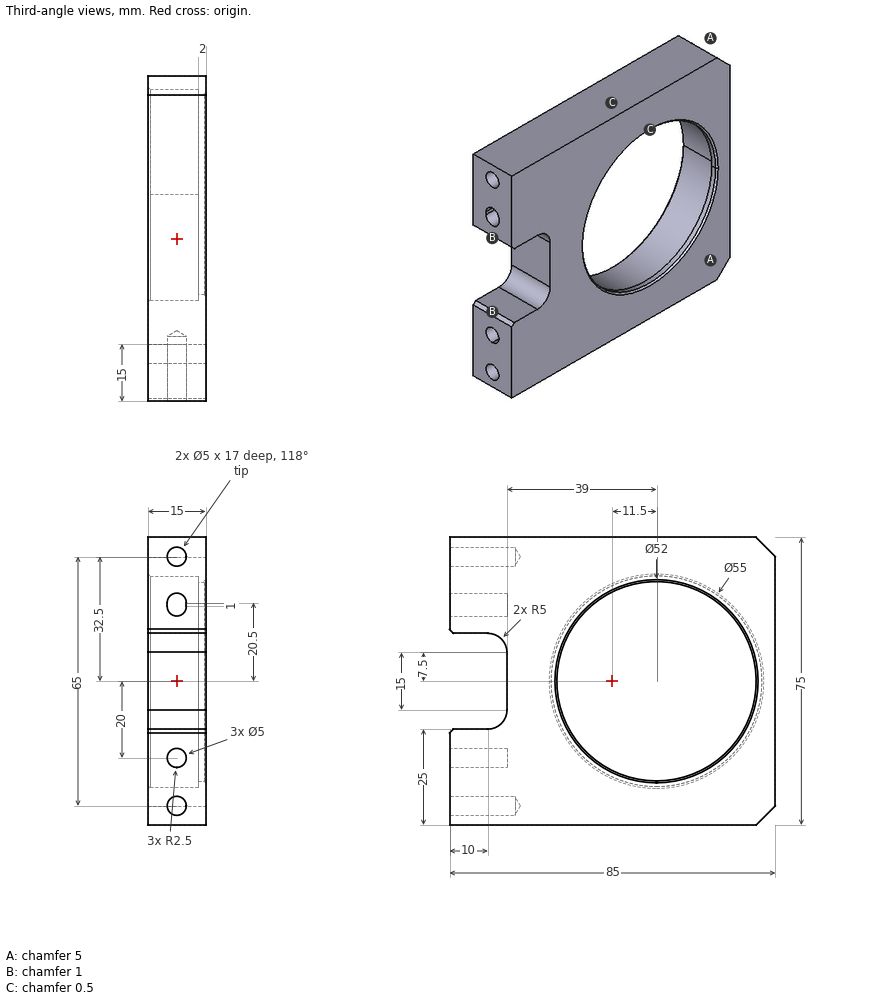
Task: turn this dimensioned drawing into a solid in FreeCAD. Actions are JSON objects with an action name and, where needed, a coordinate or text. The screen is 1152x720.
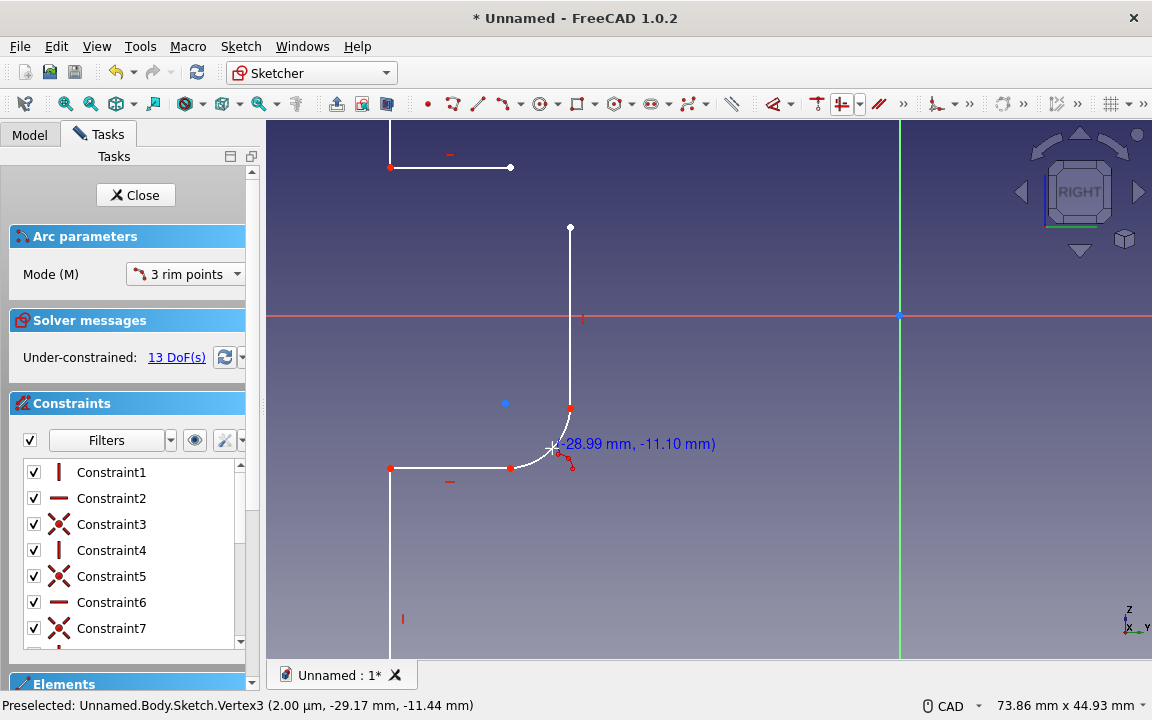
{"action": "left_click", "coordinate": [510, 168]}
{"action": "left_click", "coordinate": [570, 228]}
{"action": "left_click", "coordinate": [552, 183]}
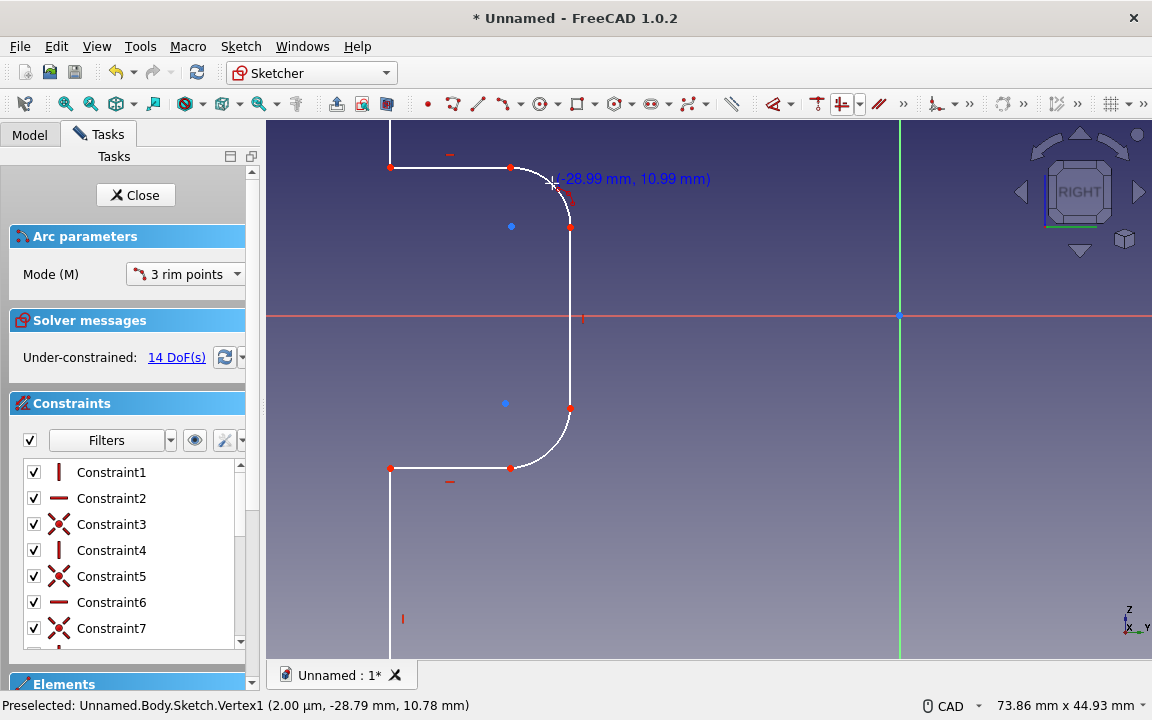
{"action": "left_click", "coordinate": [540, 104]}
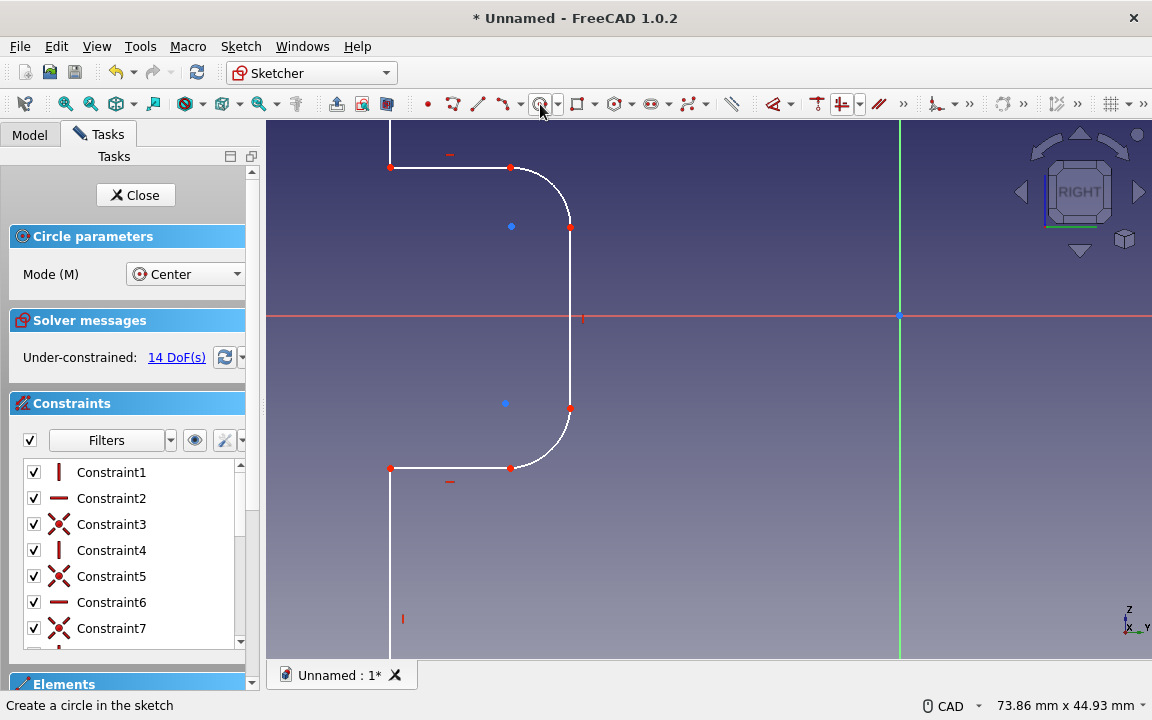
{"action": "scroll", "coordinate": [490, 432], "scroll_direction": "down", "scroll_amount": 5}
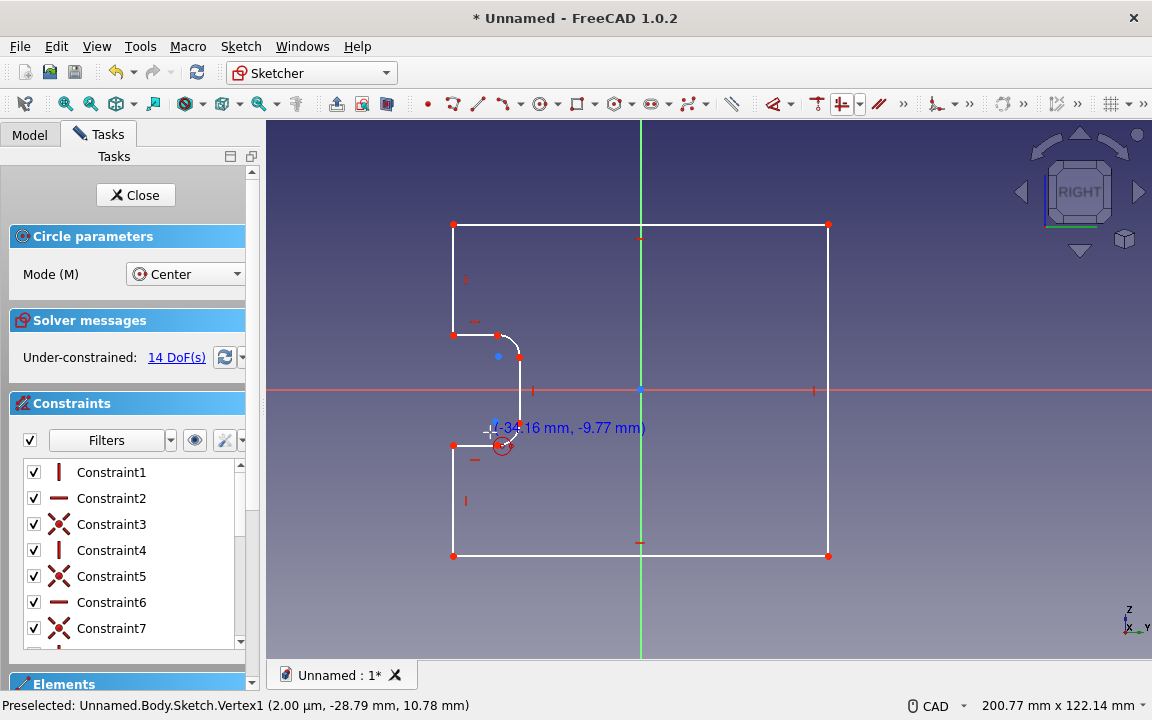
{"action": "left_click", "coordinate": [692, 390]}
{"action": "mouse_move", "coordinate": [777, 304]}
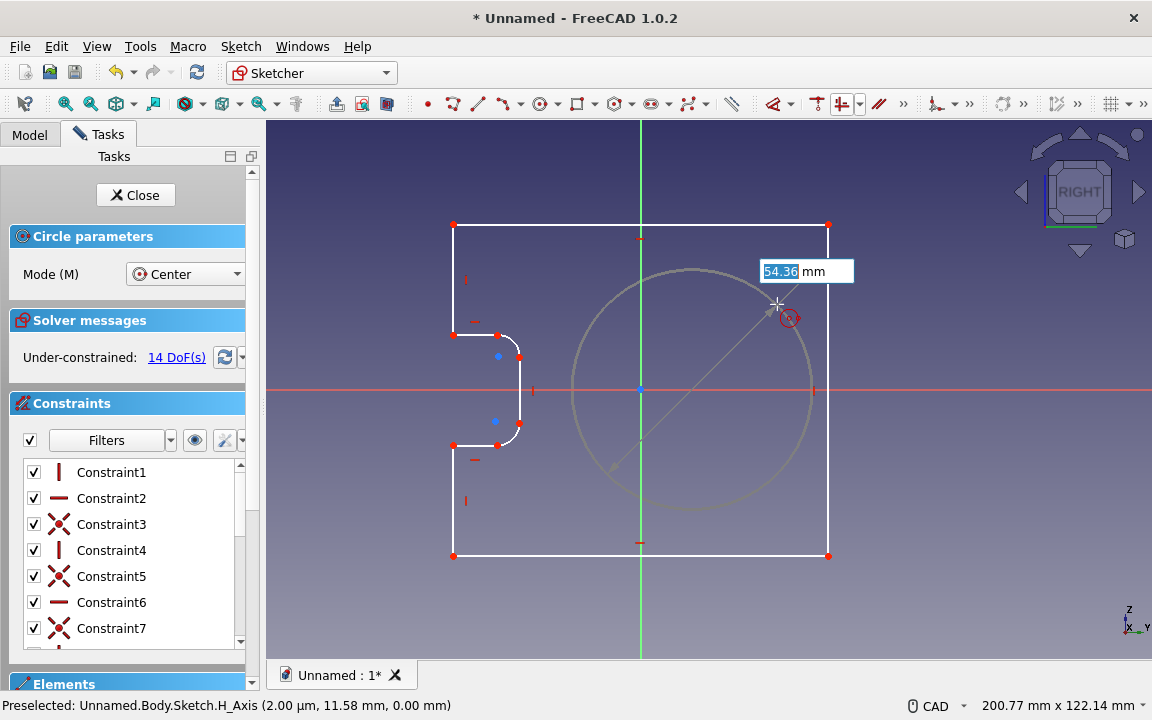
{"action": "type", "text": "55"}
{"action": "key", "text": "Return"}
{"action": "key", "text": "Escape"}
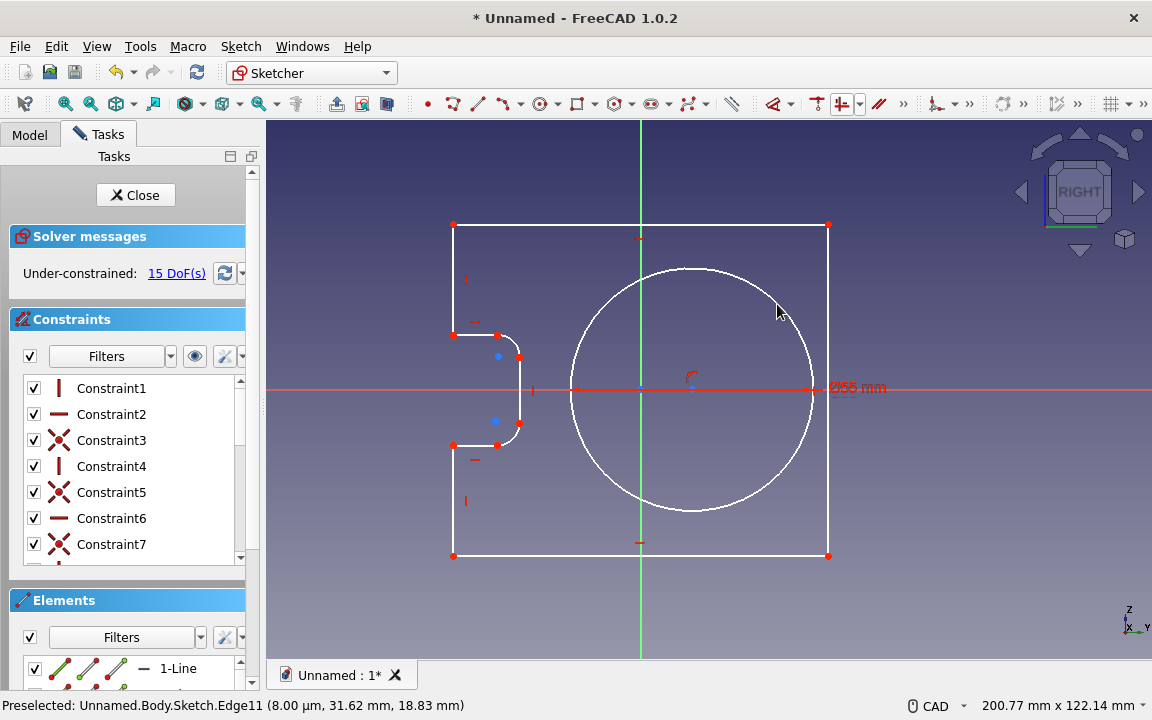
{"action": "left_click", "coordinate": [520, 377]}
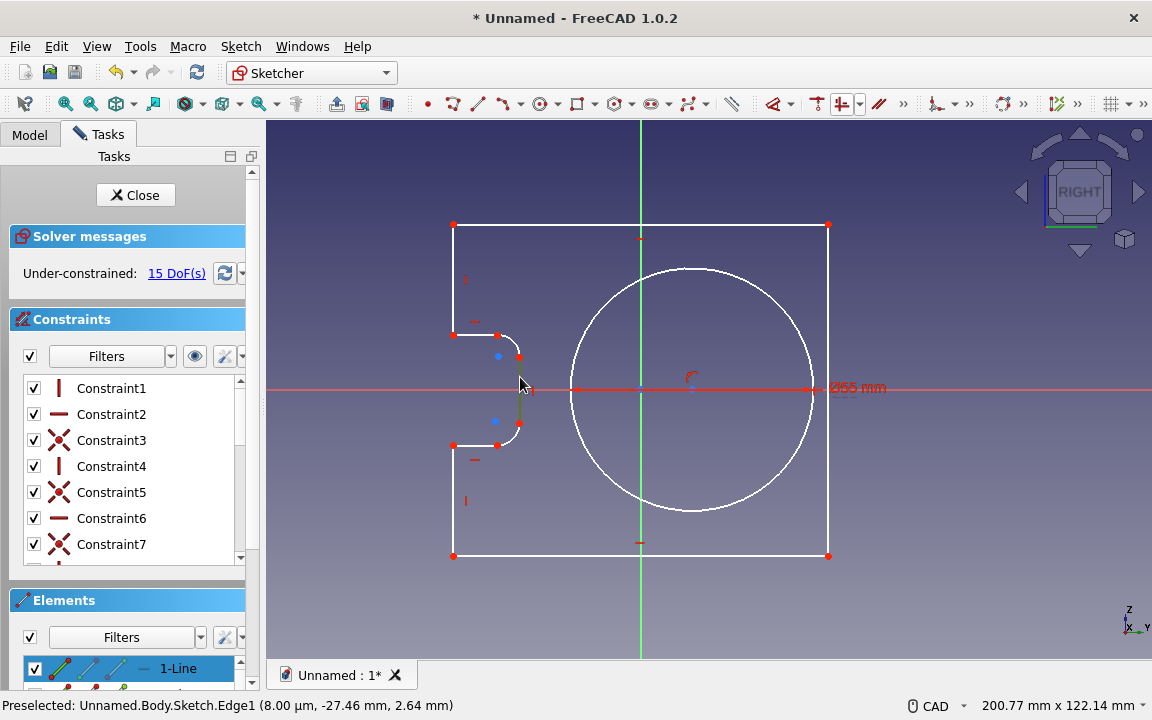
{"action": "scroll", "coordinate": [507, 443], "scroll_direction": "up", "scroll_amount": 2}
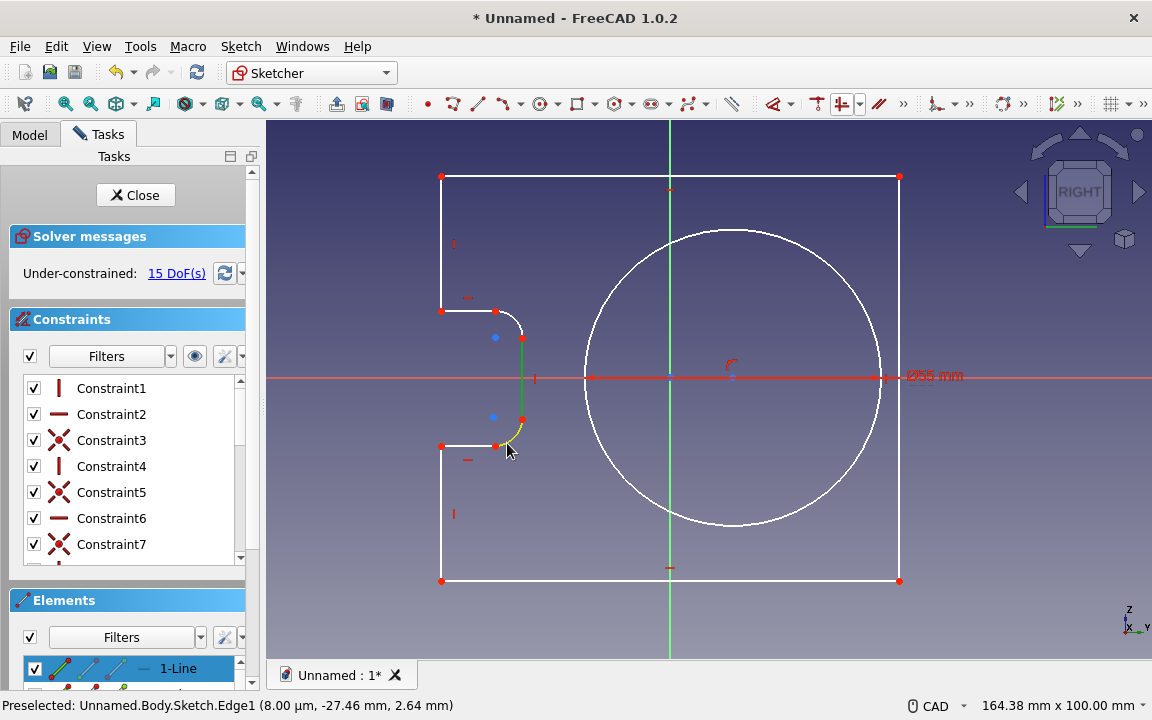
{"action": "left_click", "coordinate": [507, 442]}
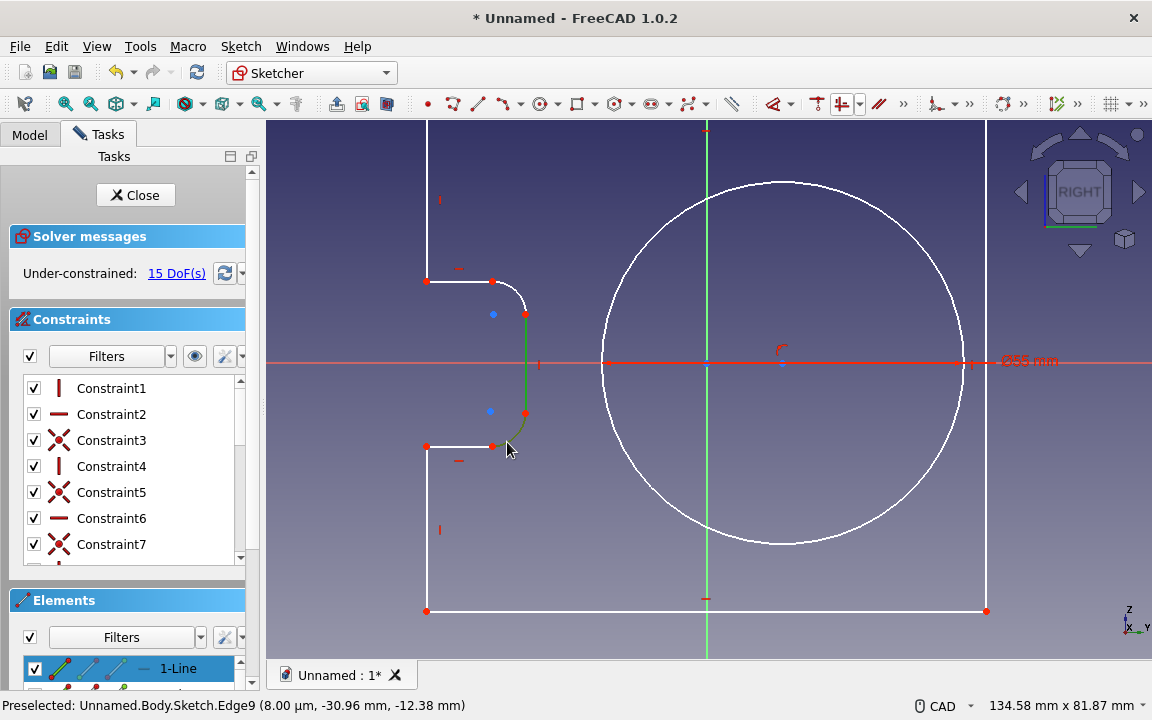
{"action": "key", "text": "t"}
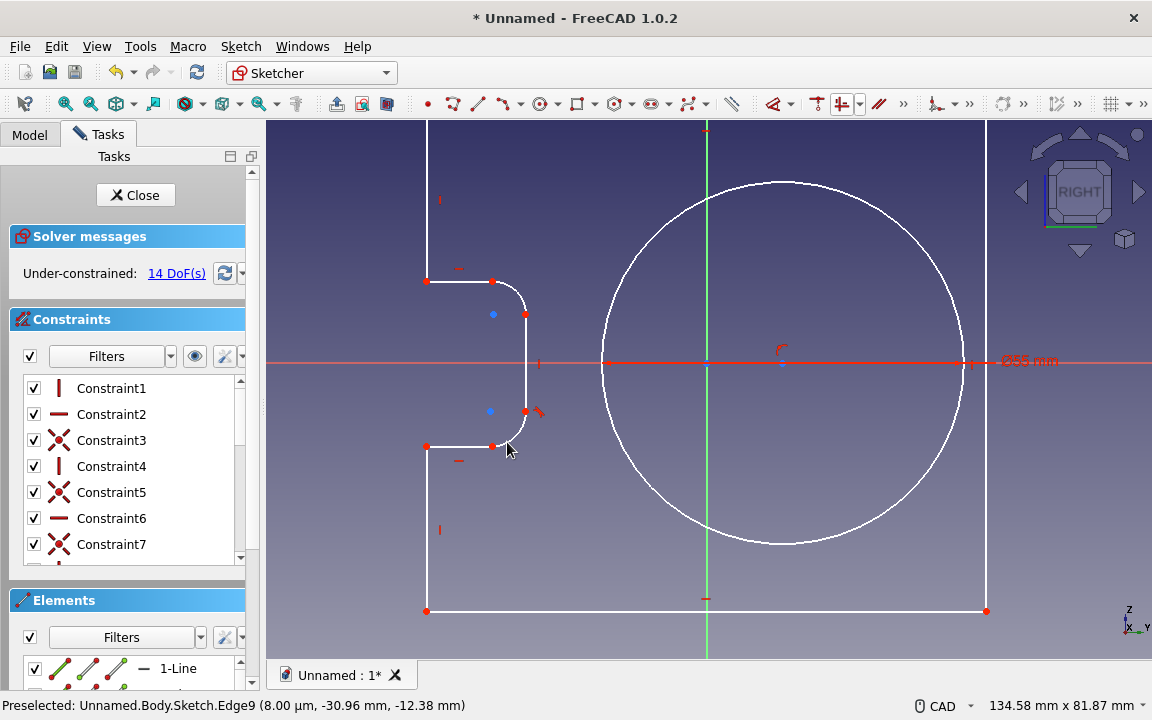
{"action": "left_click", "coordinate": [526, 344]}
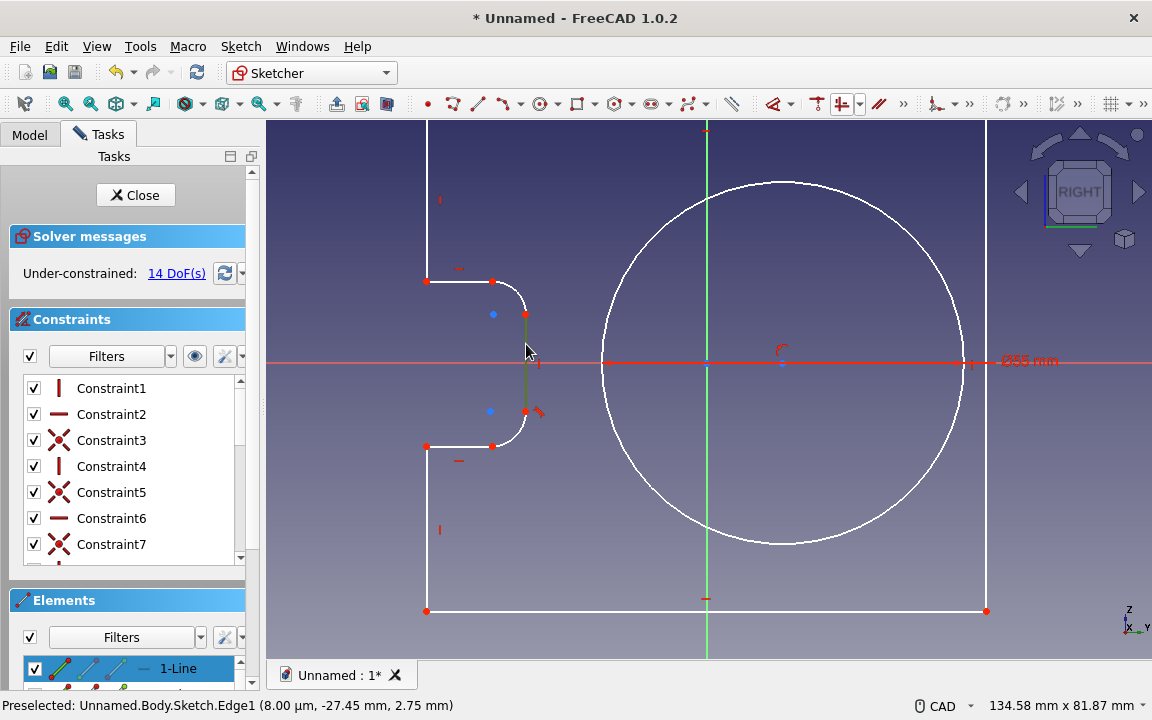
{"action": "left_click", "coordinate": [522, 300]}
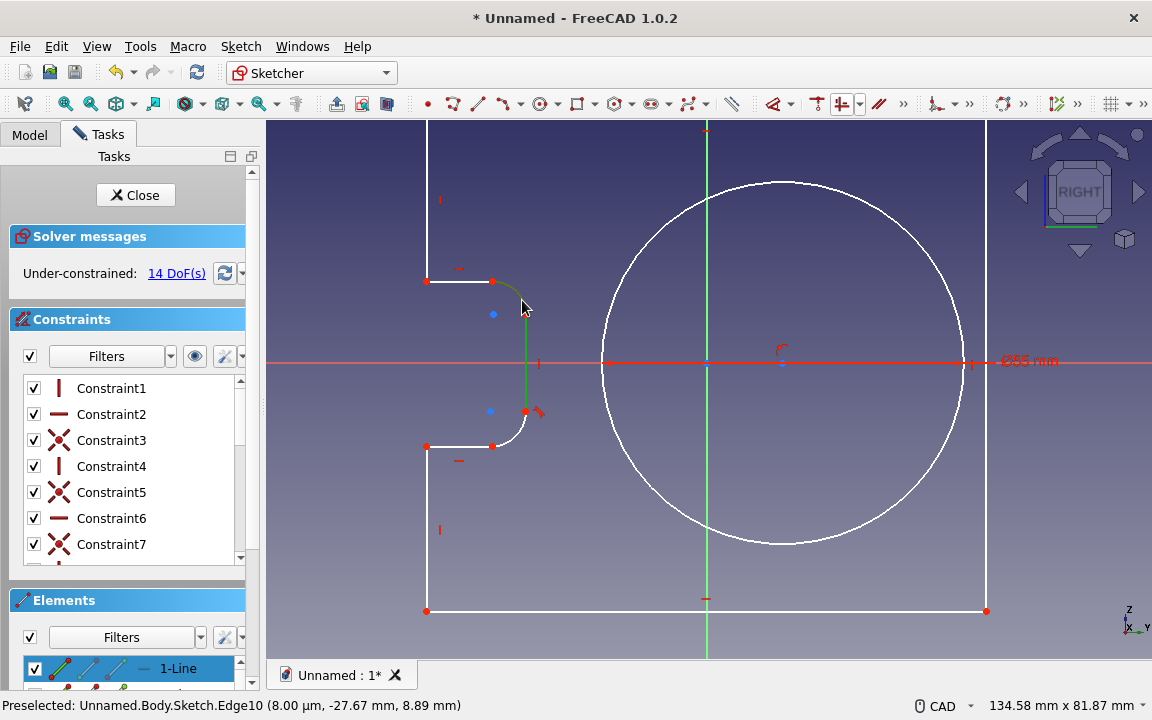
{"action": "key", "text": "t"}